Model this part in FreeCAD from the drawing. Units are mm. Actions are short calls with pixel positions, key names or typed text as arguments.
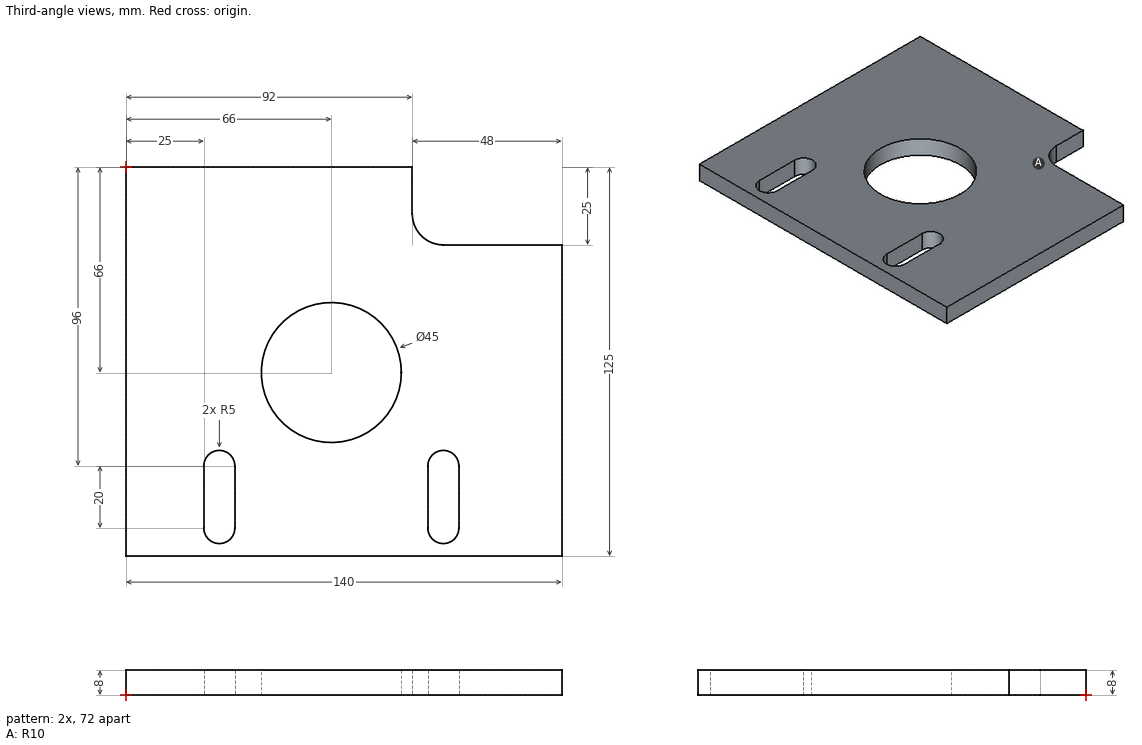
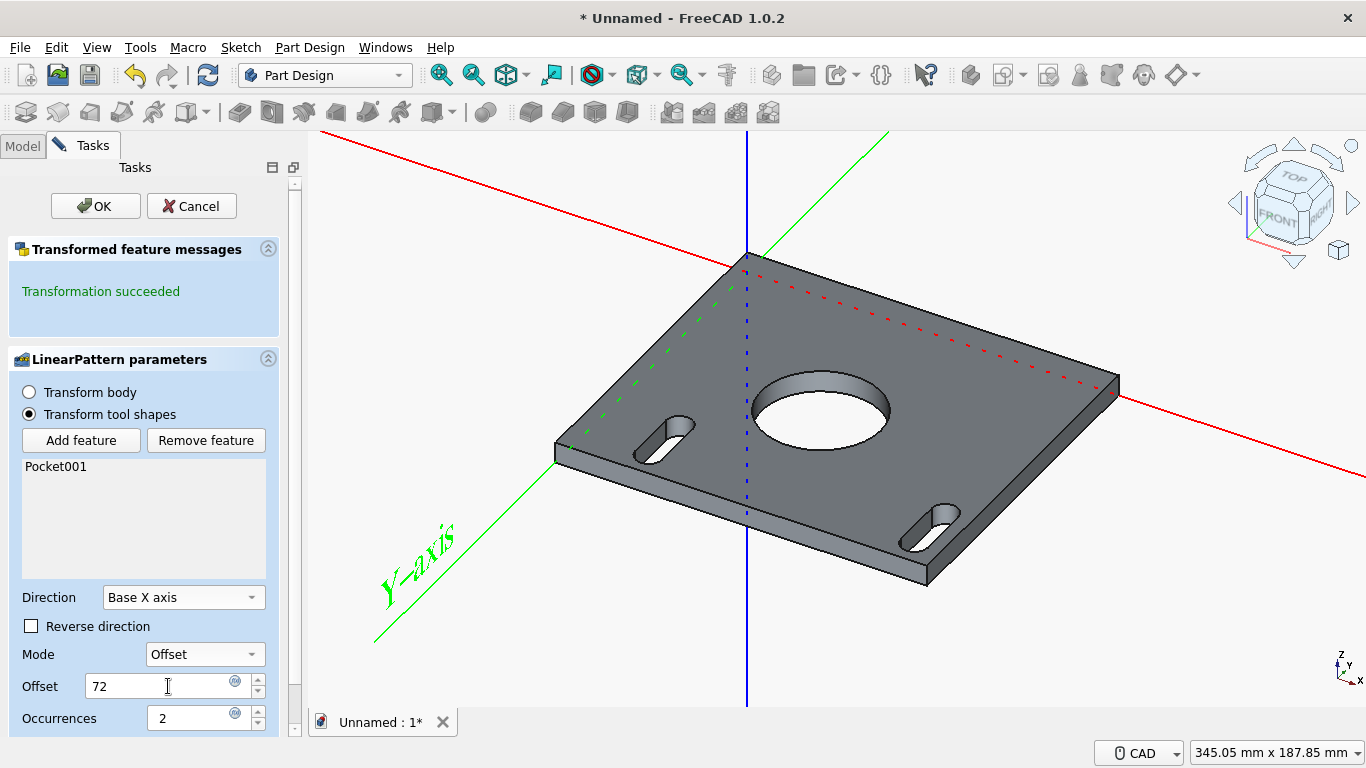
triple_click(198, 718)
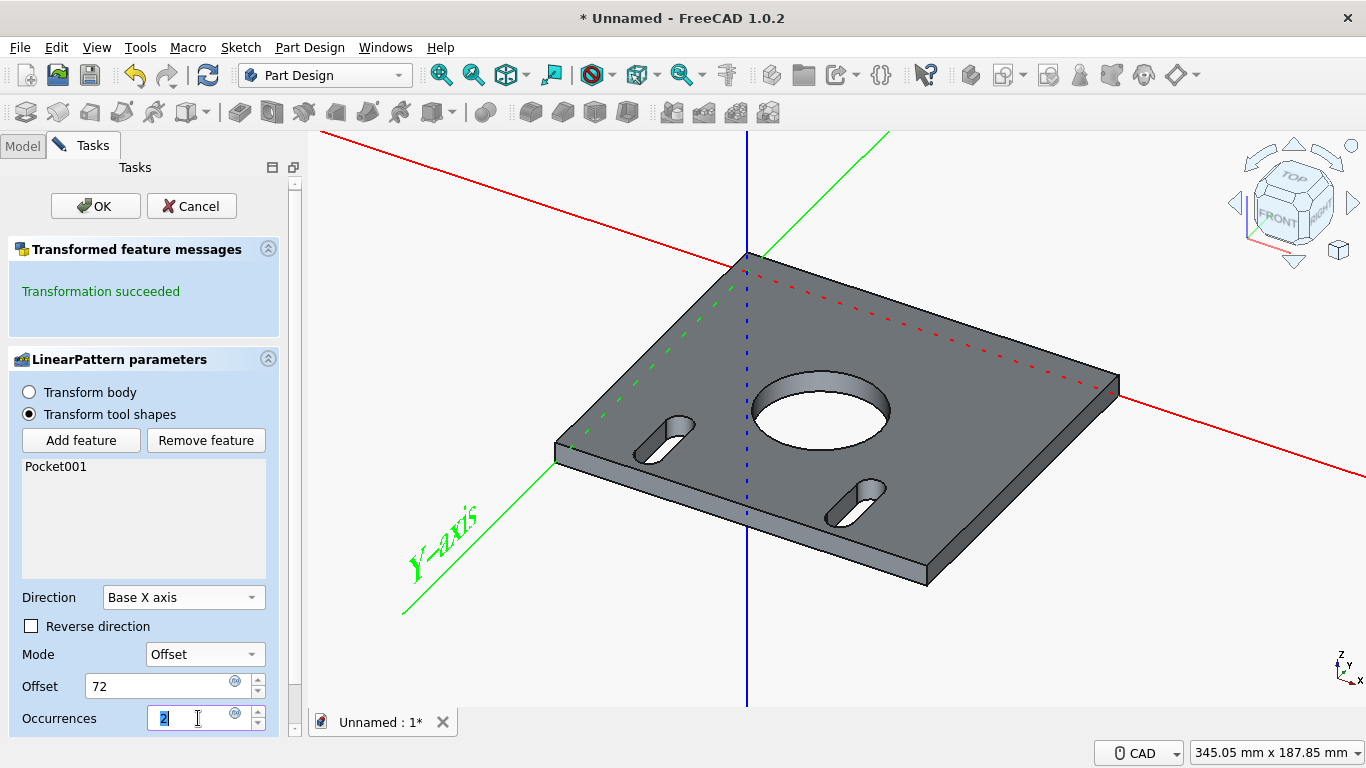
text(2)
key(Tab)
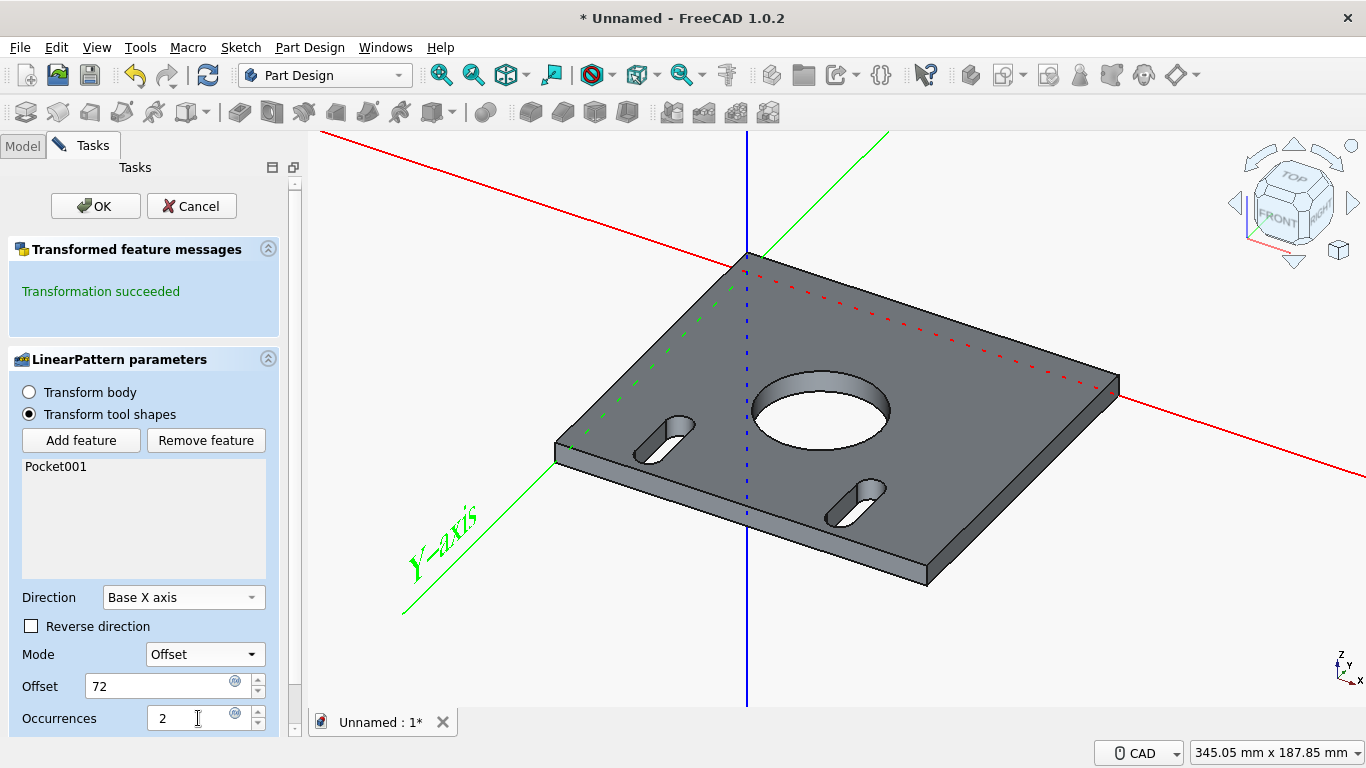
click(96, 206)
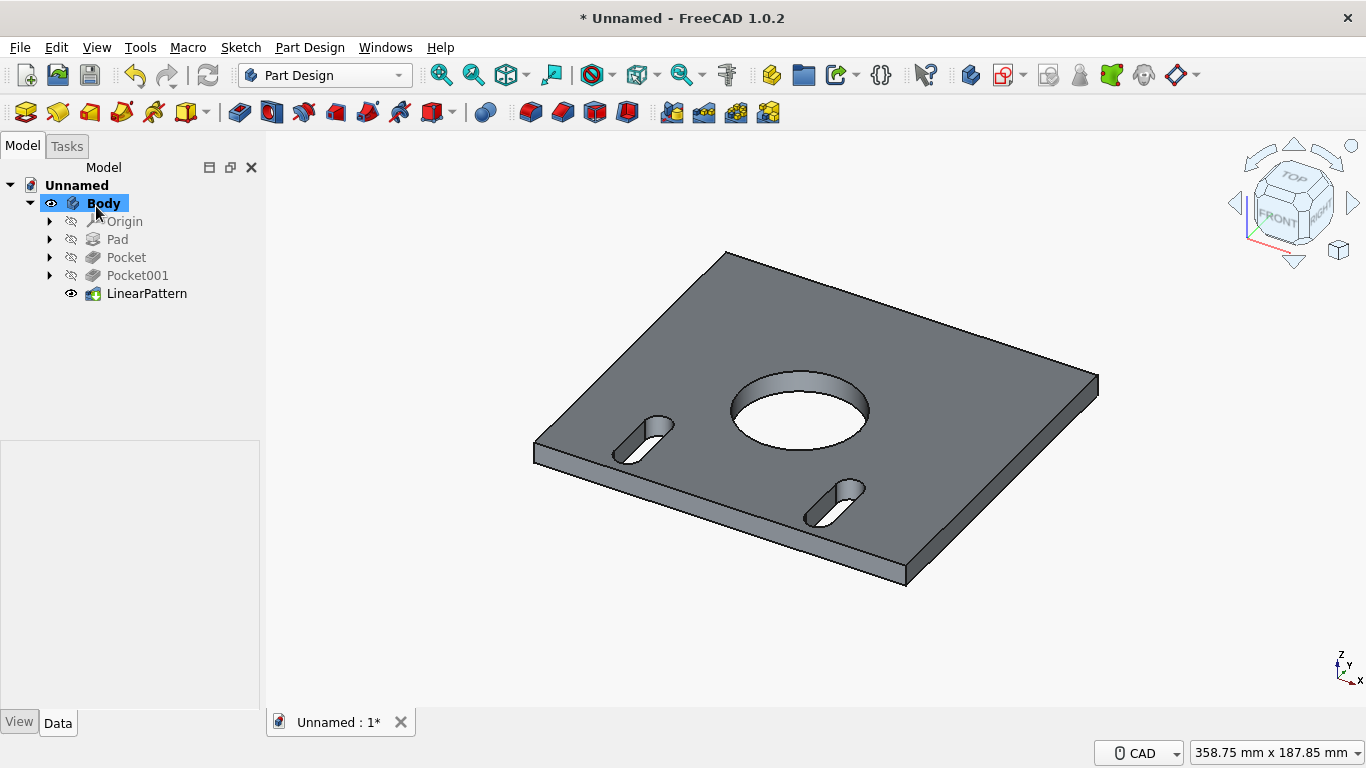
click(977, 389)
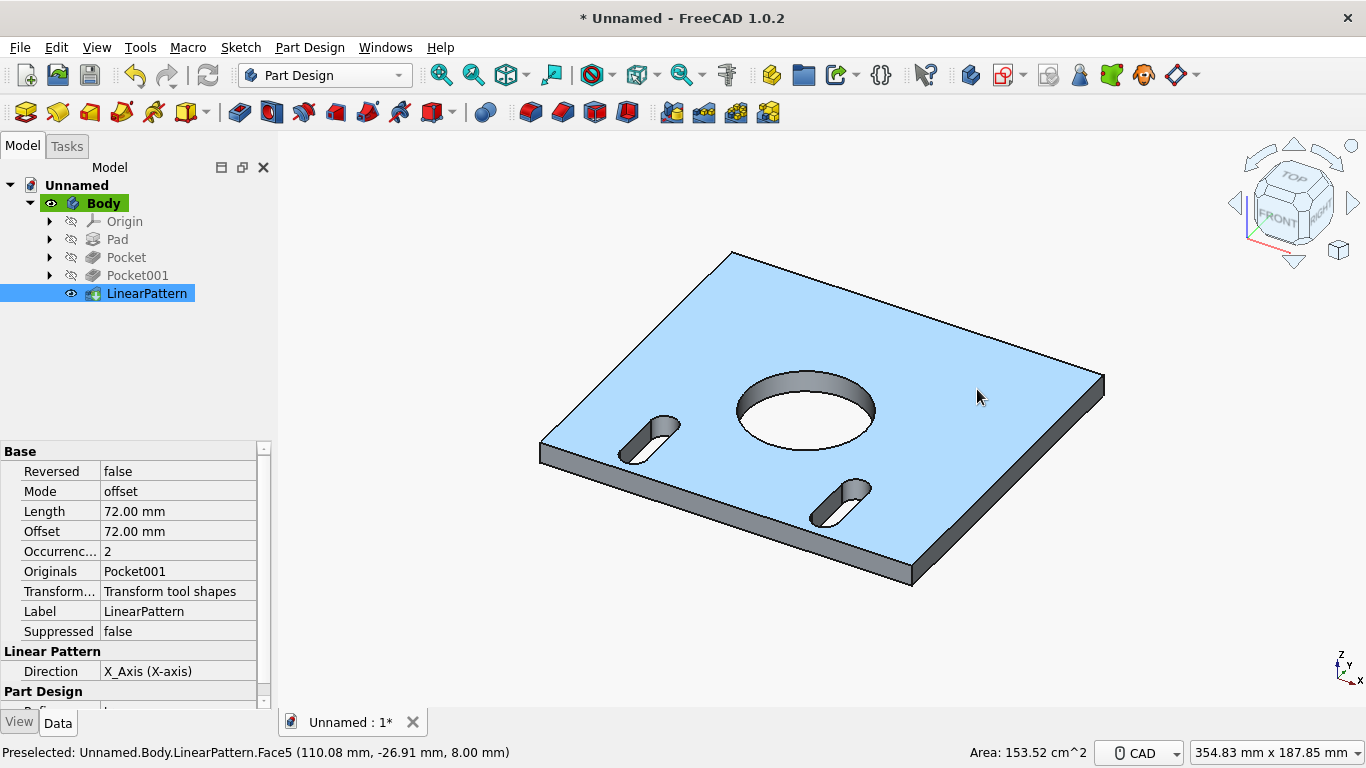
click(1004, 76)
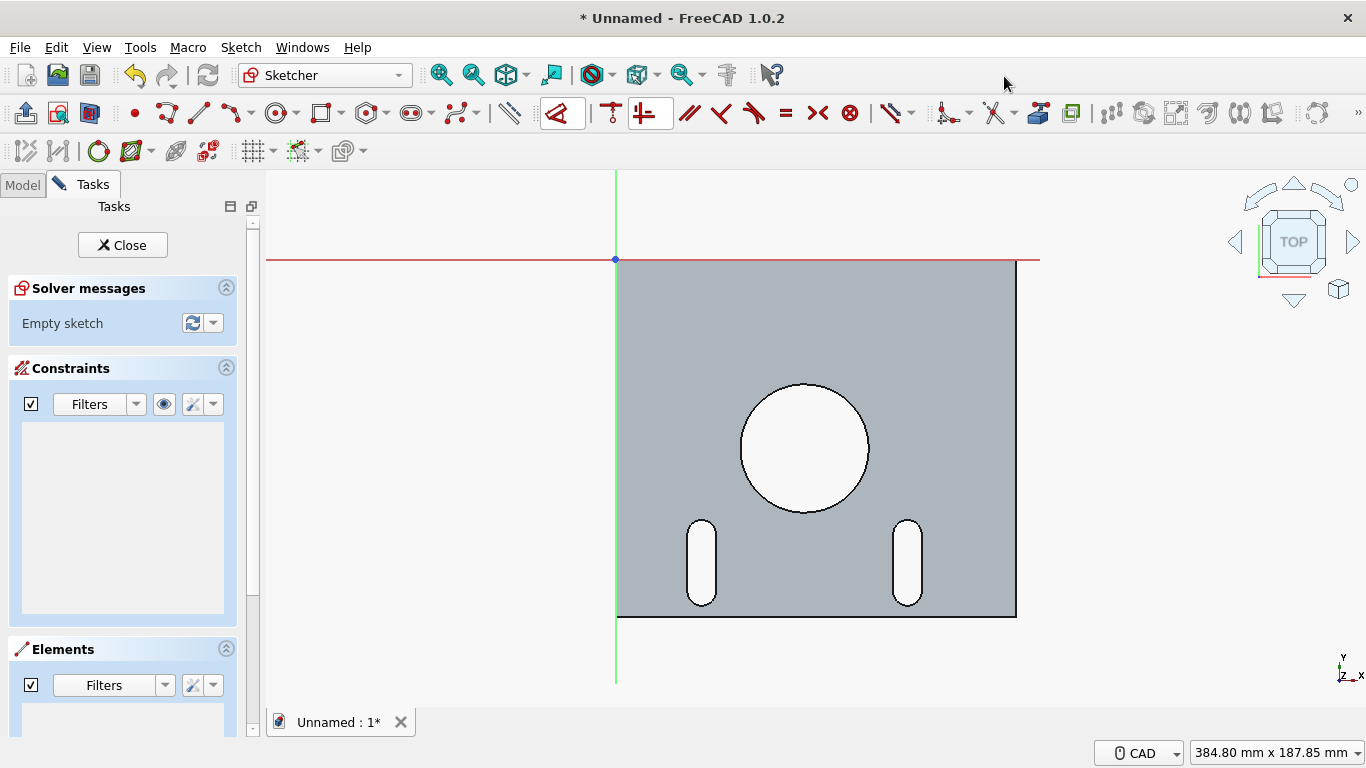
scroll(998, 259, up, 8)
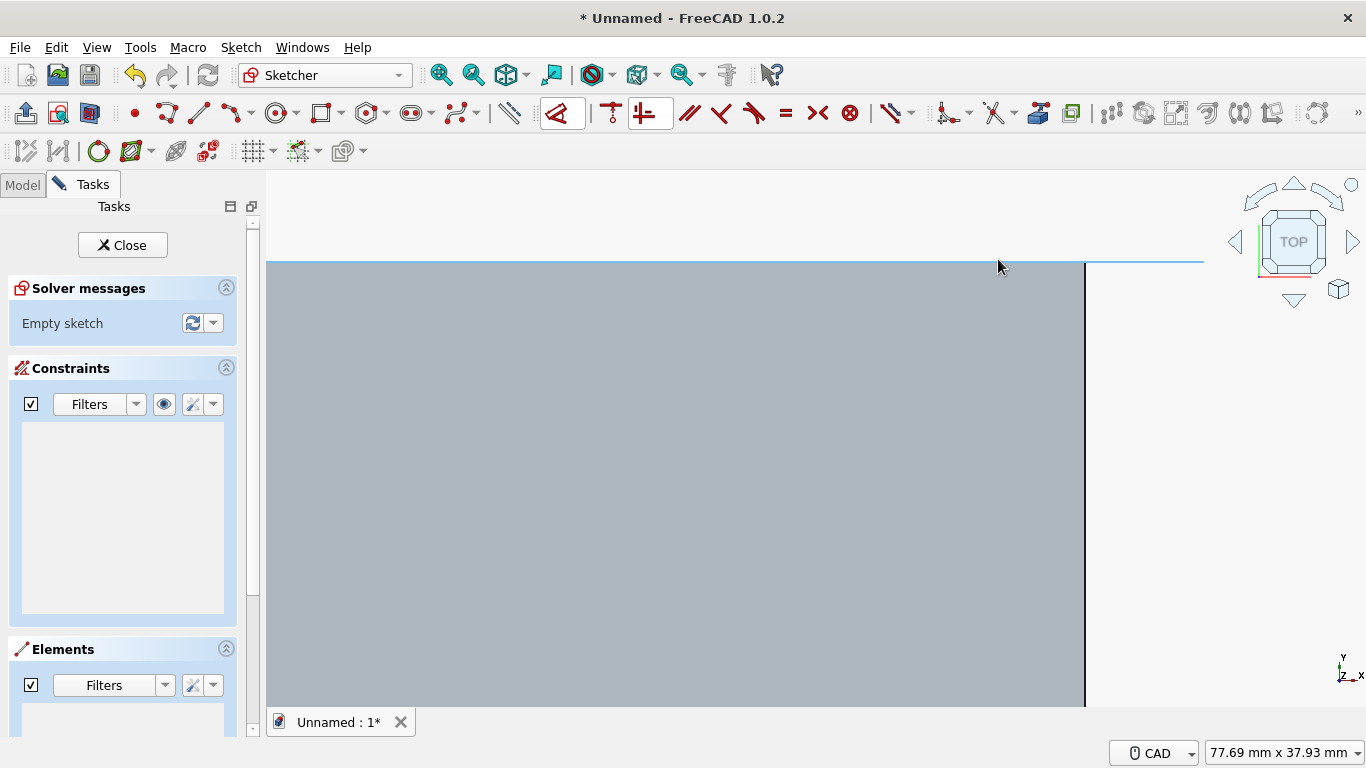
key(g)
key(r)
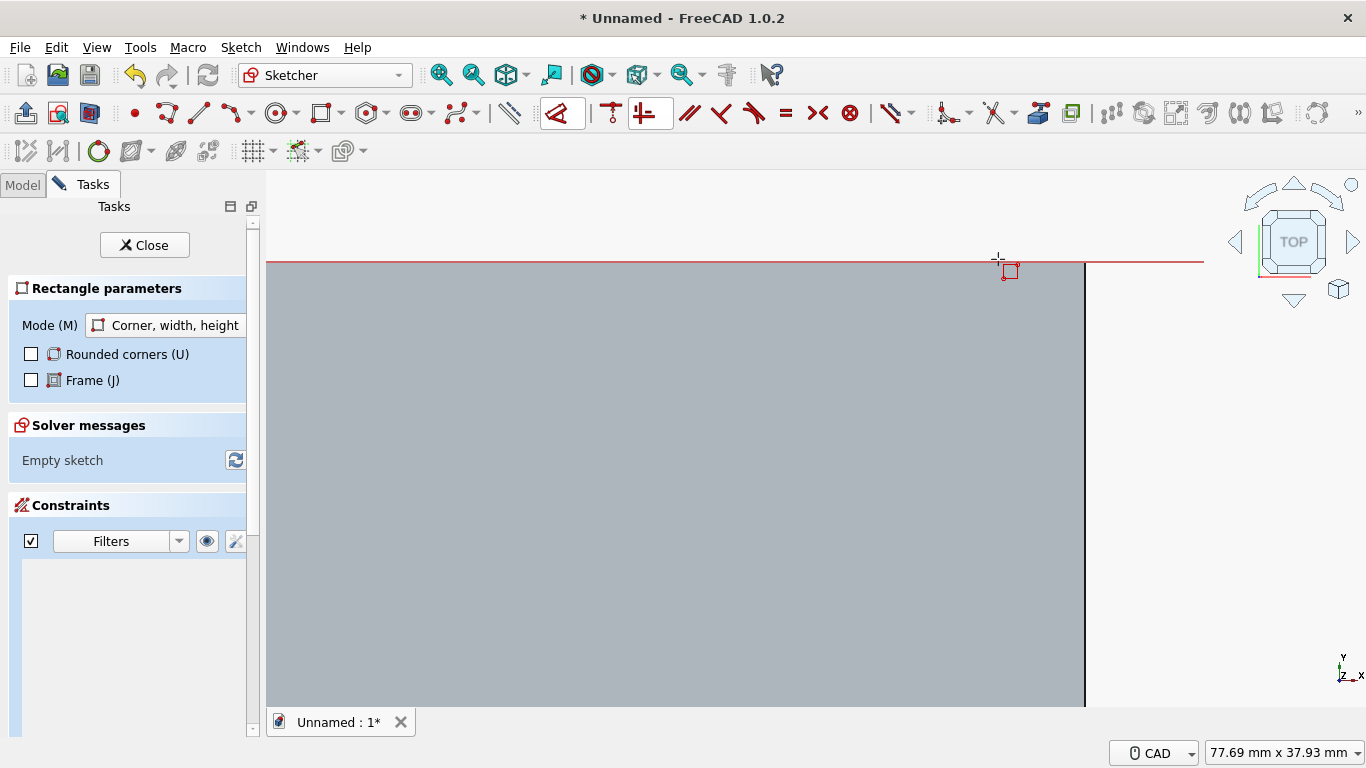
click(405, 262)
move(1085, 616)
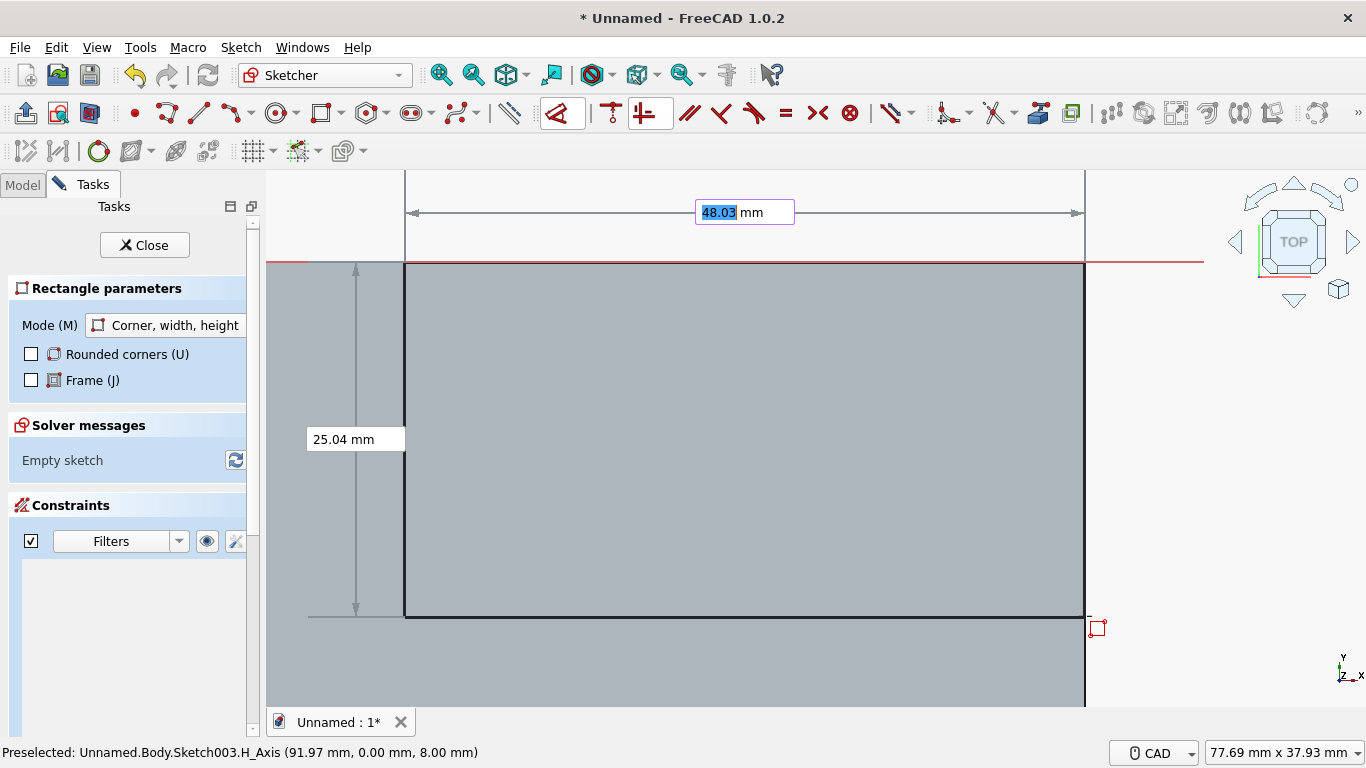
text(48)
key(Tab)
text(25)
key(Return)
key(Escape)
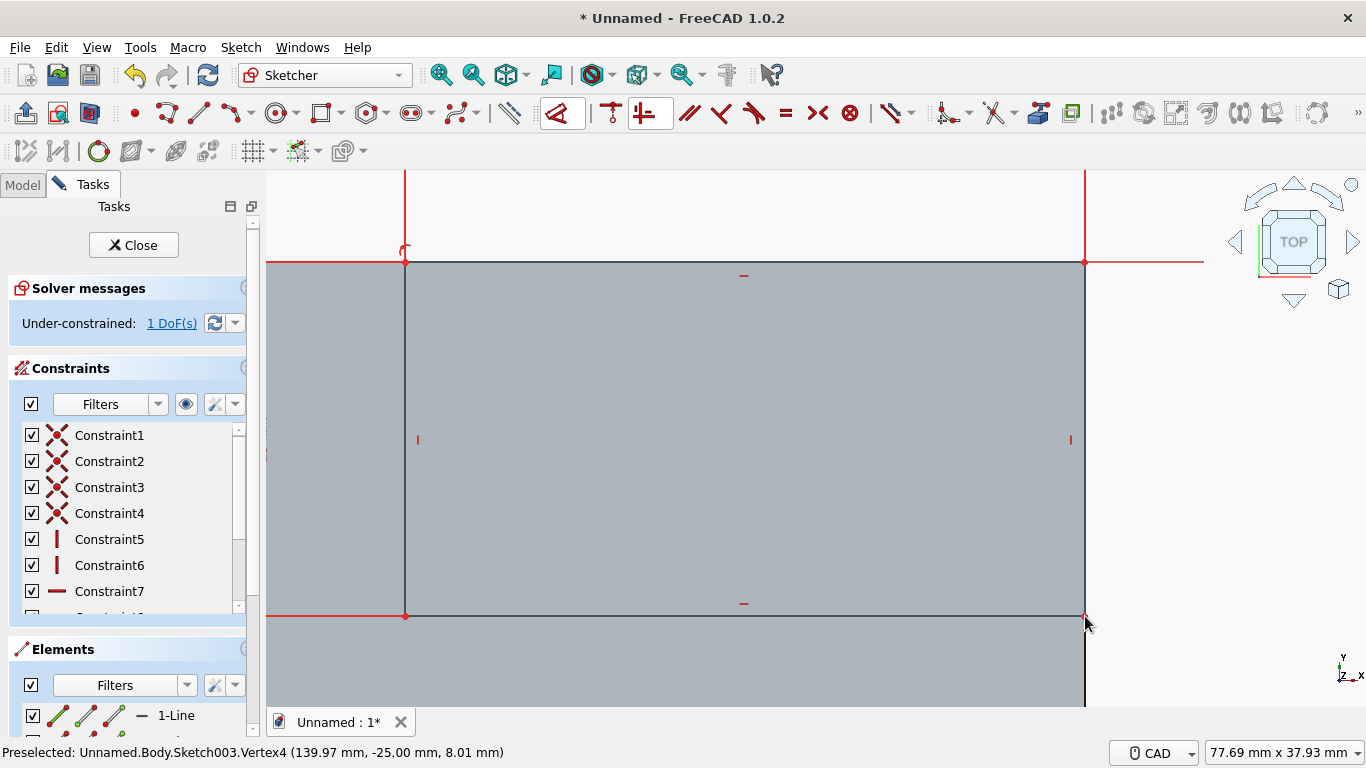
click(405, 262)